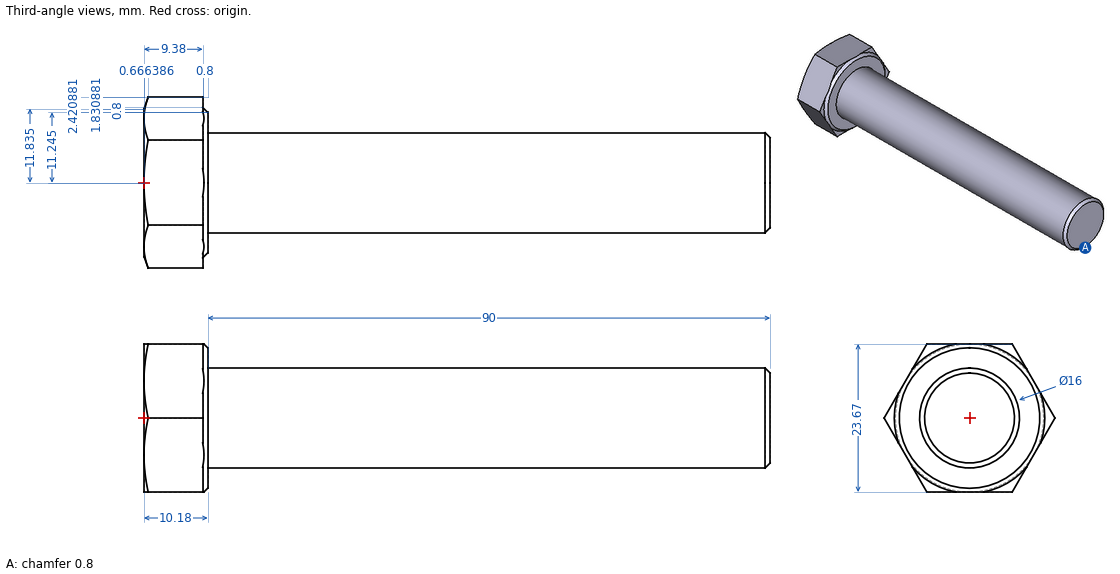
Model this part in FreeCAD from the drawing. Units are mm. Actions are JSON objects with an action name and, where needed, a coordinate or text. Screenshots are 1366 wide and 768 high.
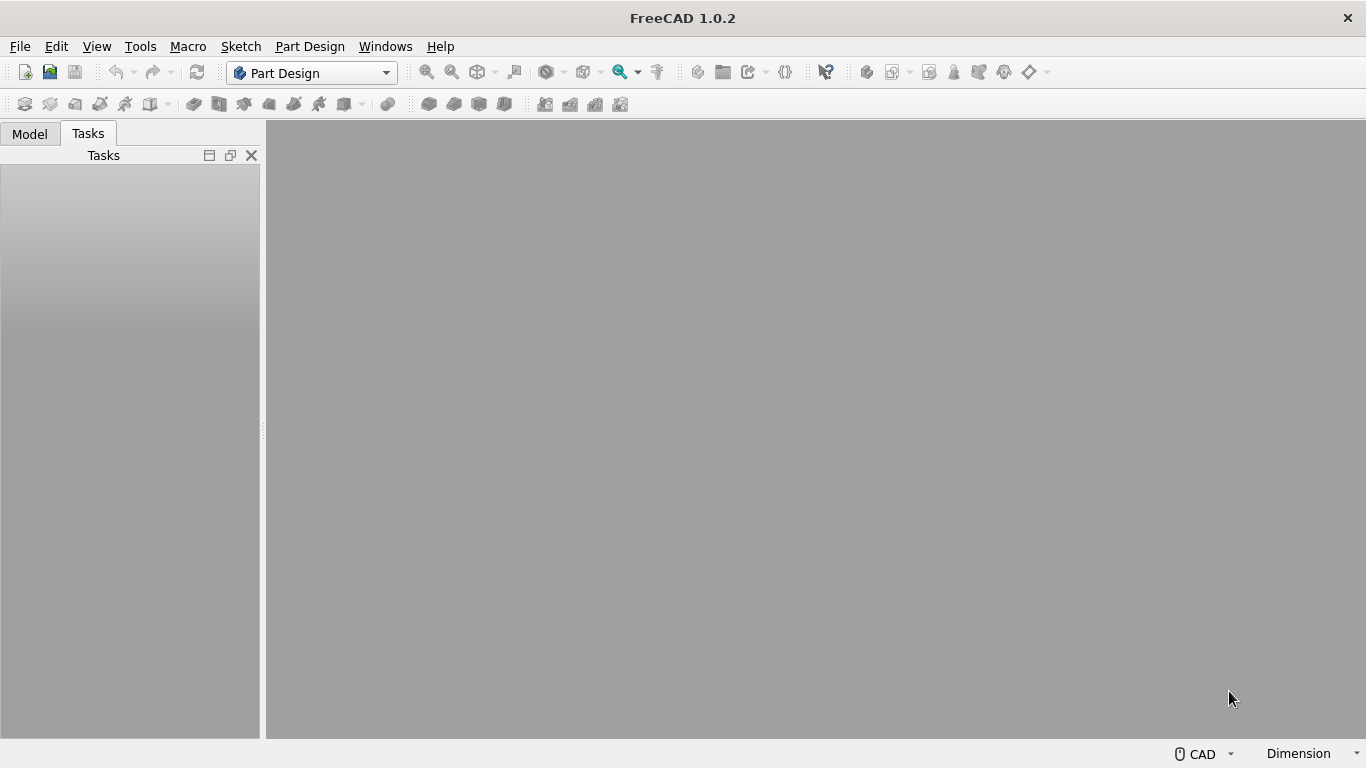
{"action": "key", "text": "ctrl+n"}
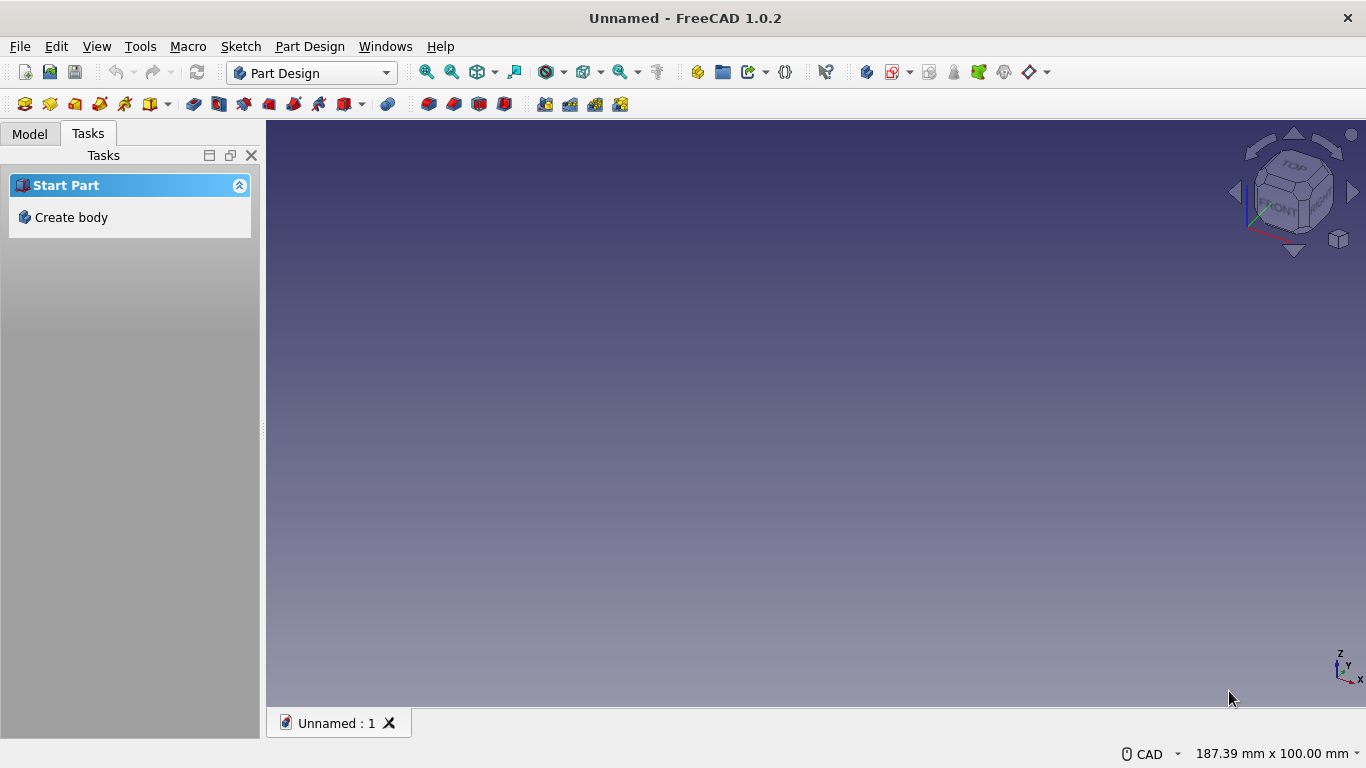
{"action": "left_click", "coordinate": [892, 72]}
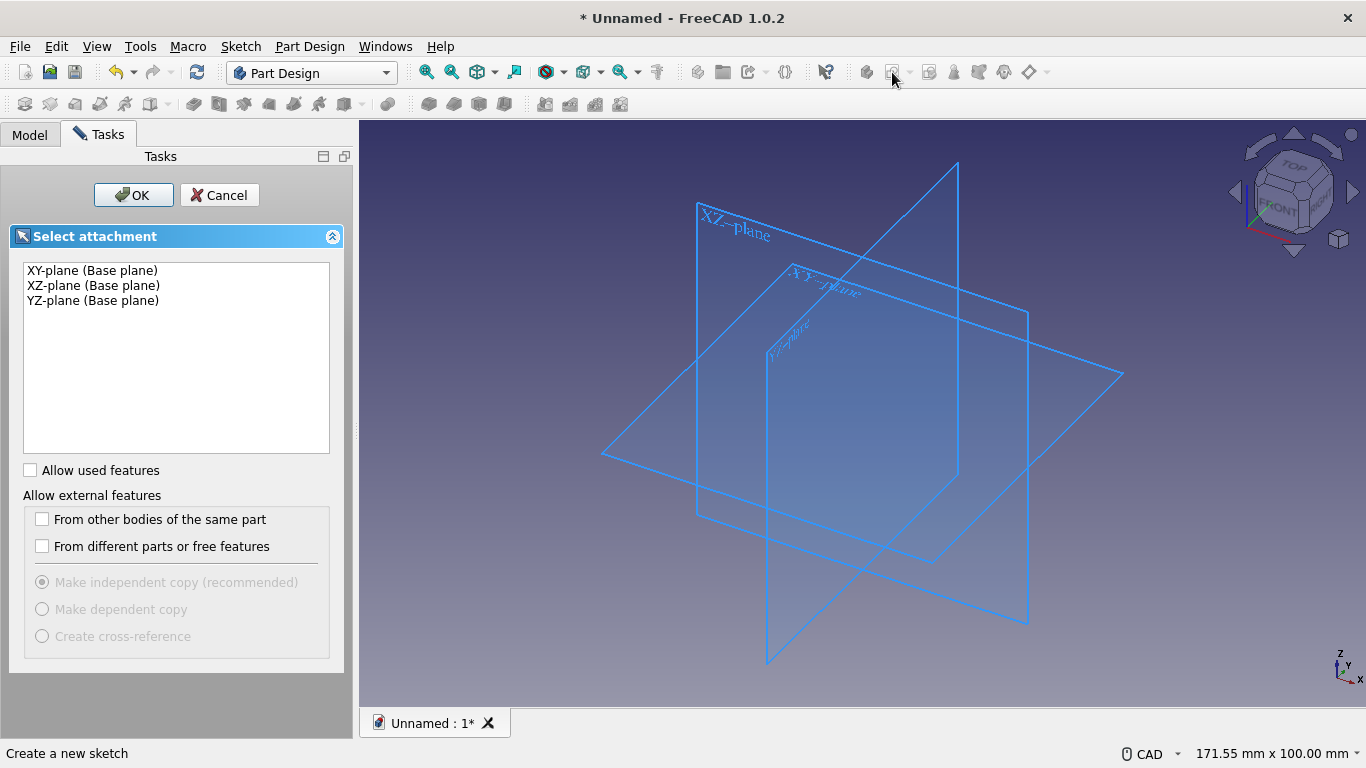
{"action": "left_click", "coordinate": [84, 300]}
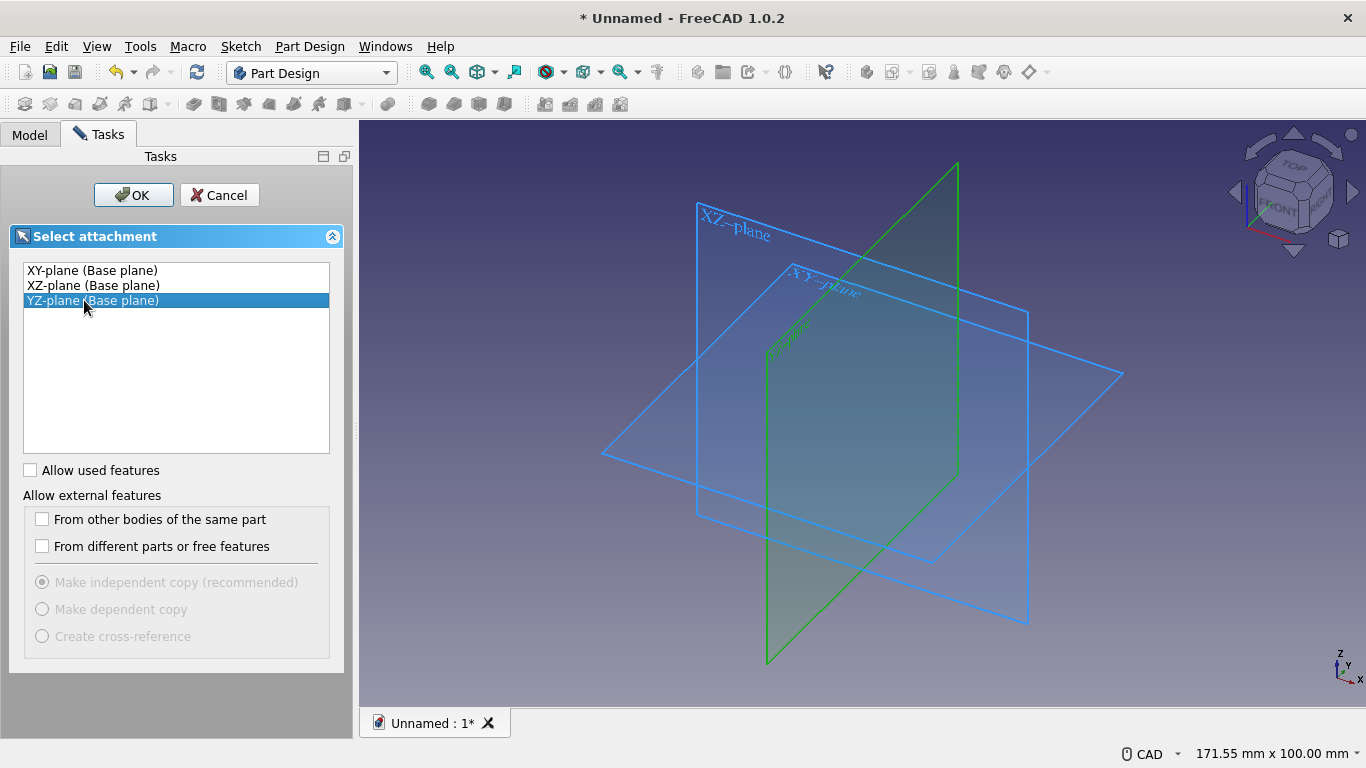
{"action": "left_click", "coordinate": [134, 195]}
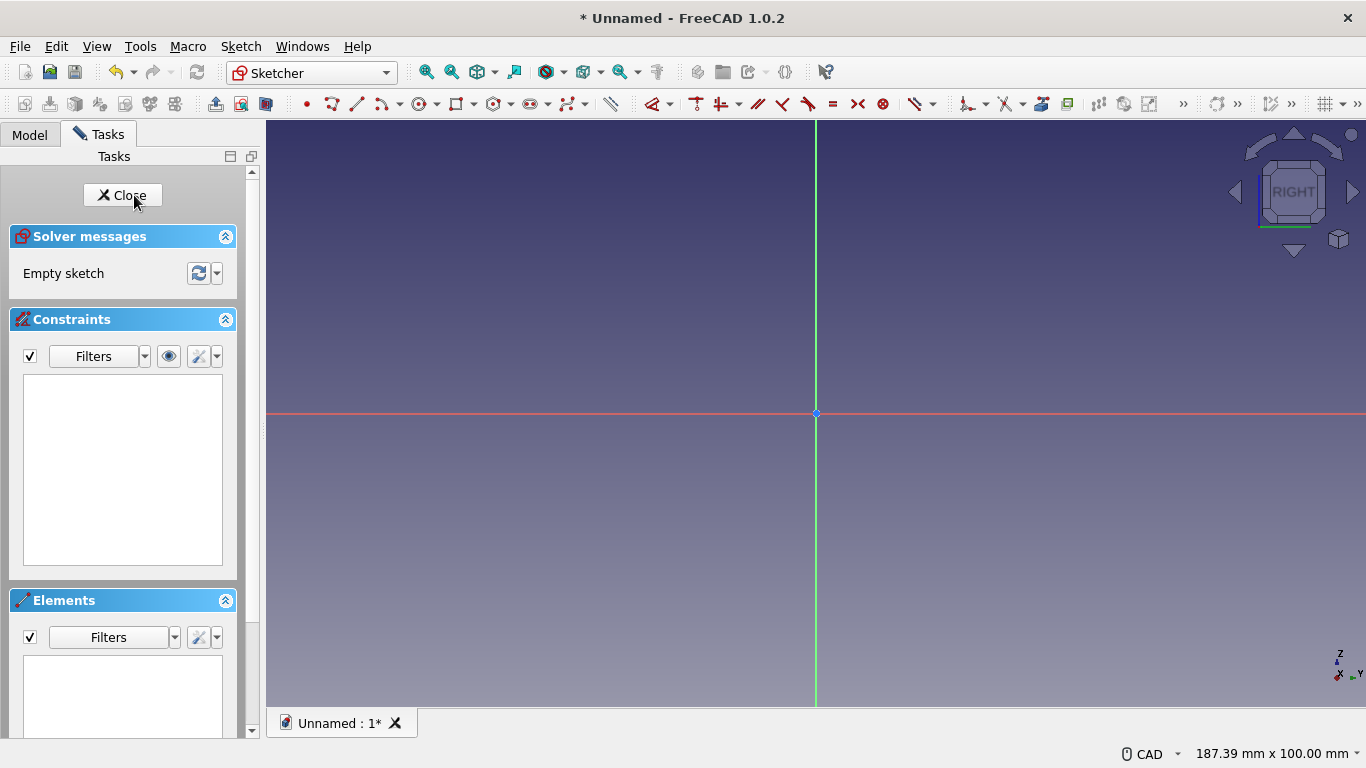
{"action": "scroll", "coordinate": [856, 414], "scroll_direction": "up", "scroll_amount": 5}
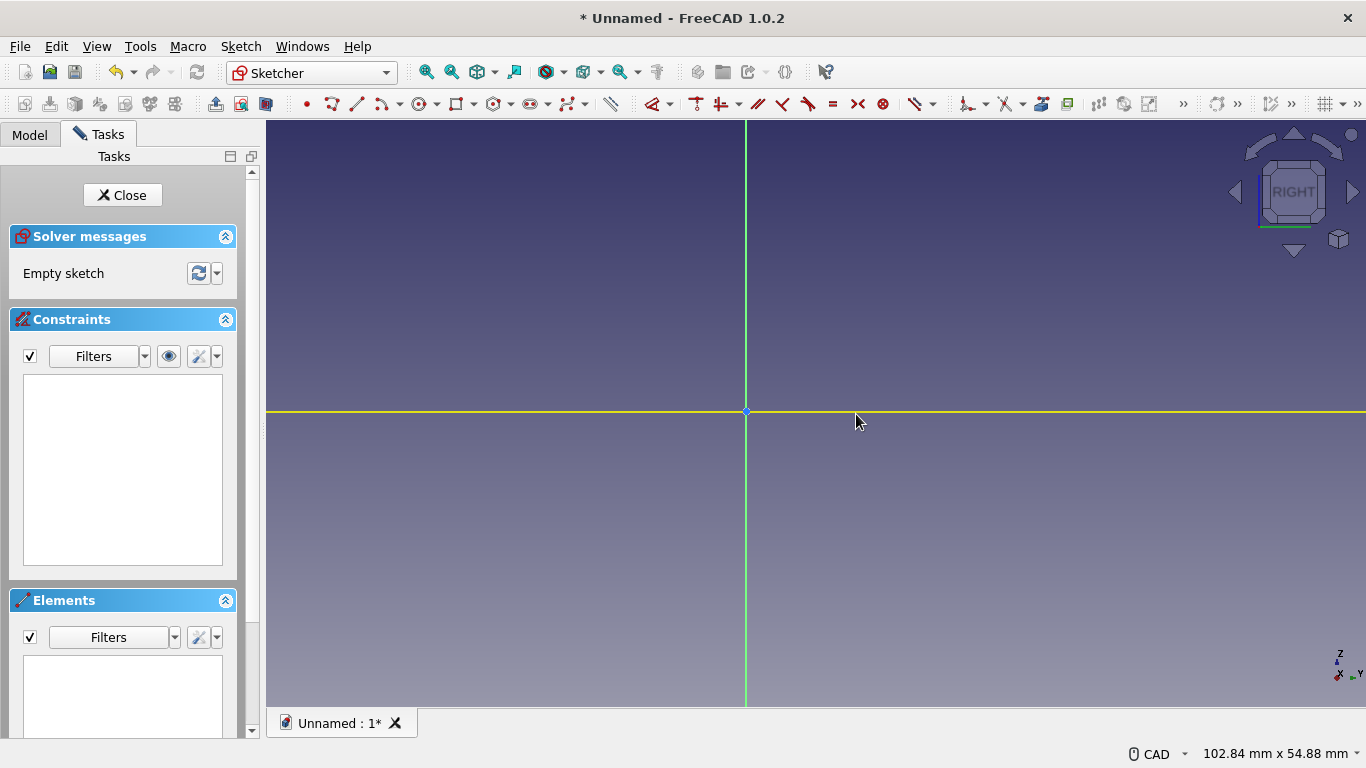
{"action": "left_click", "coordinate": [492, 104]}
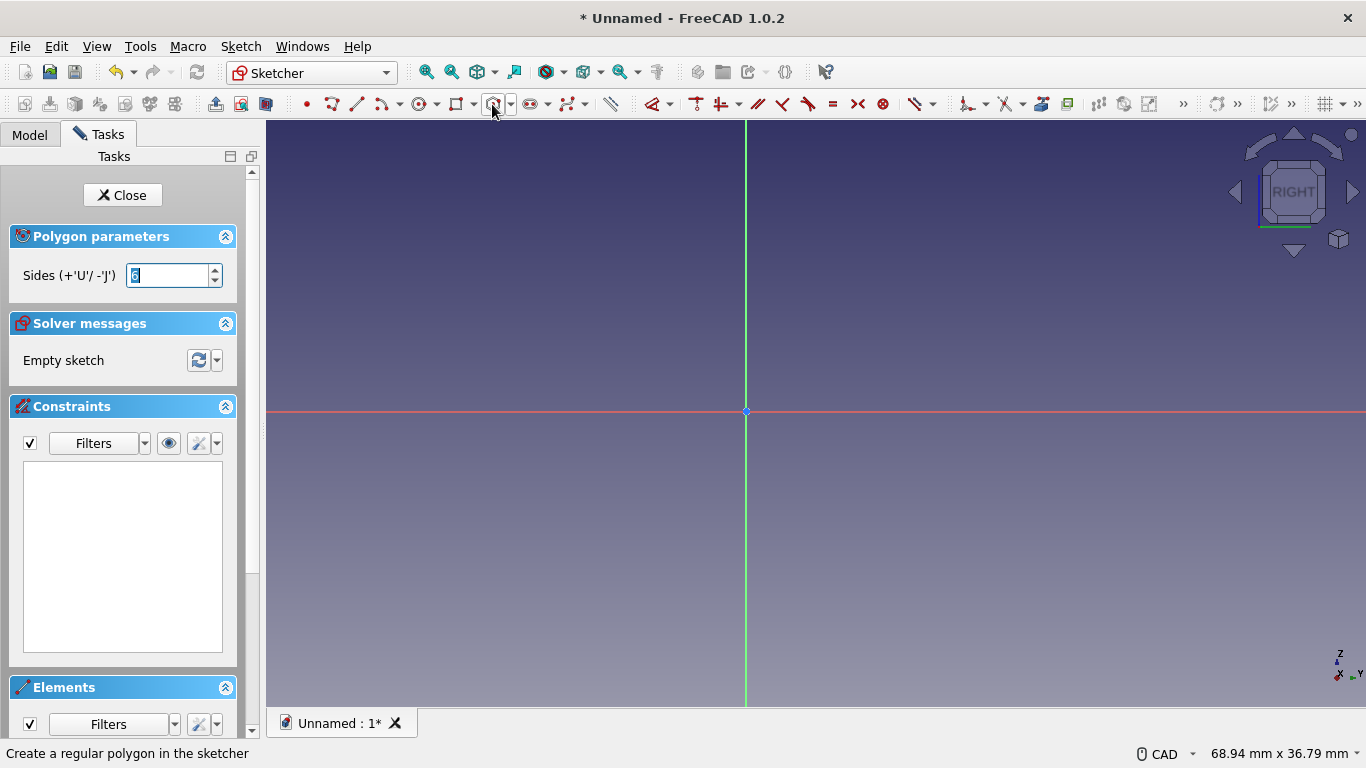
{"action": "left_click", "coordinate": [746, 412]}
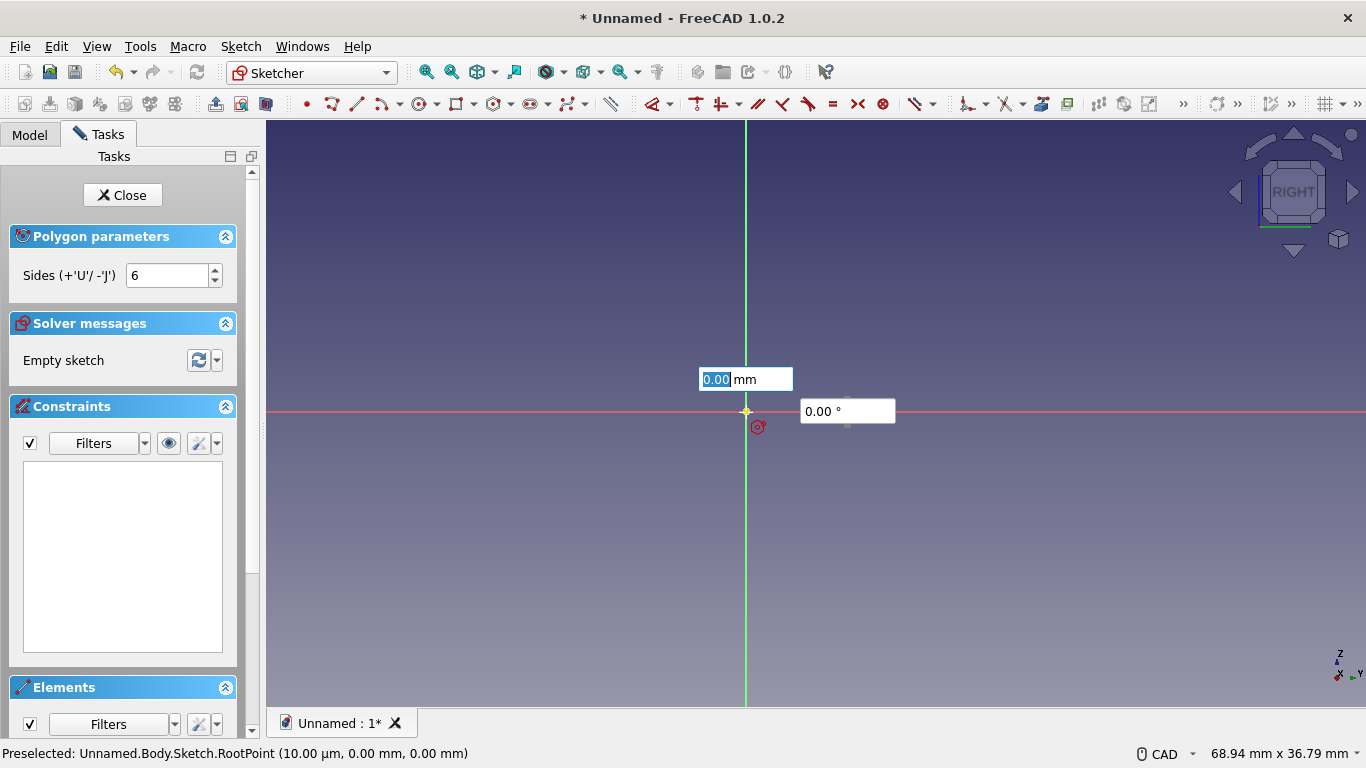
{"action": "left_click", "coordinate": [964, 412]}
{"action": "right_click", "coordinate": [964, 412]}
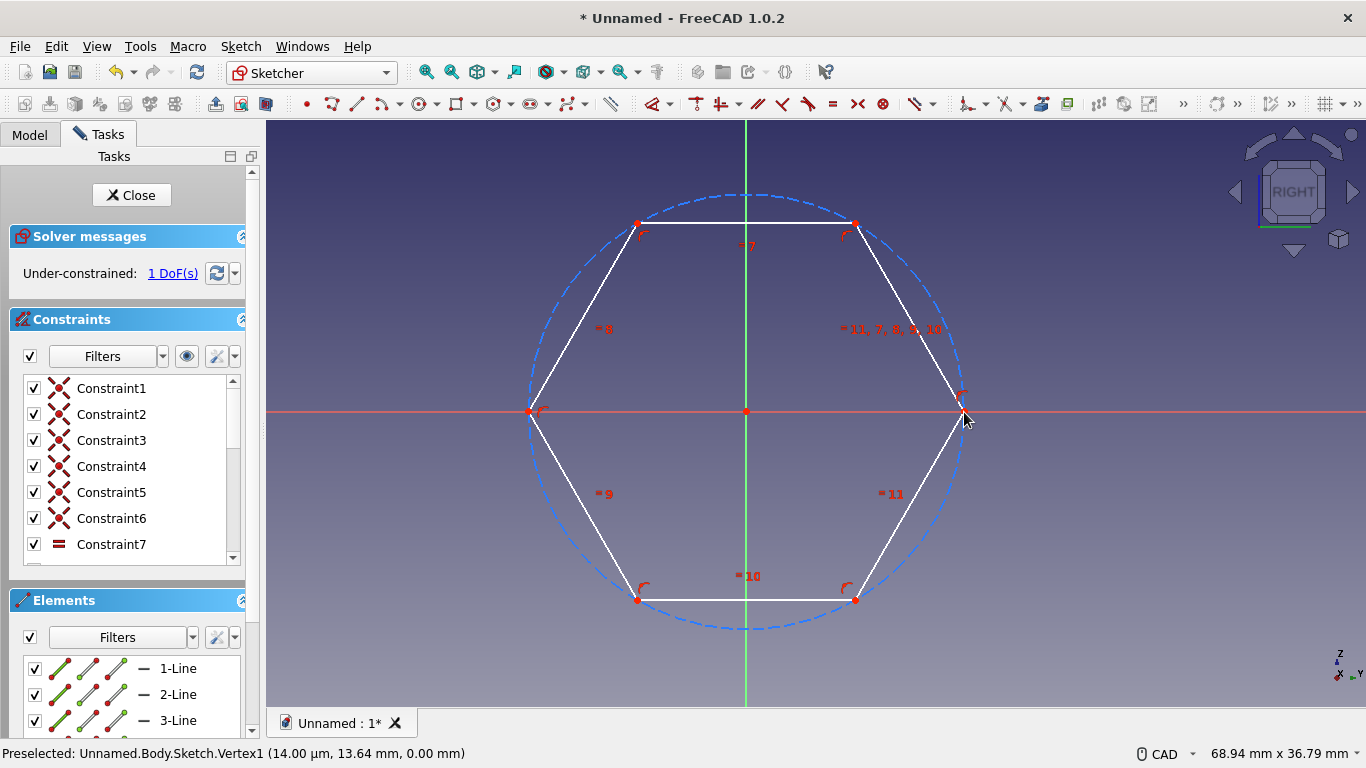
{"action": "left_click", "coordinate": [638, 600]}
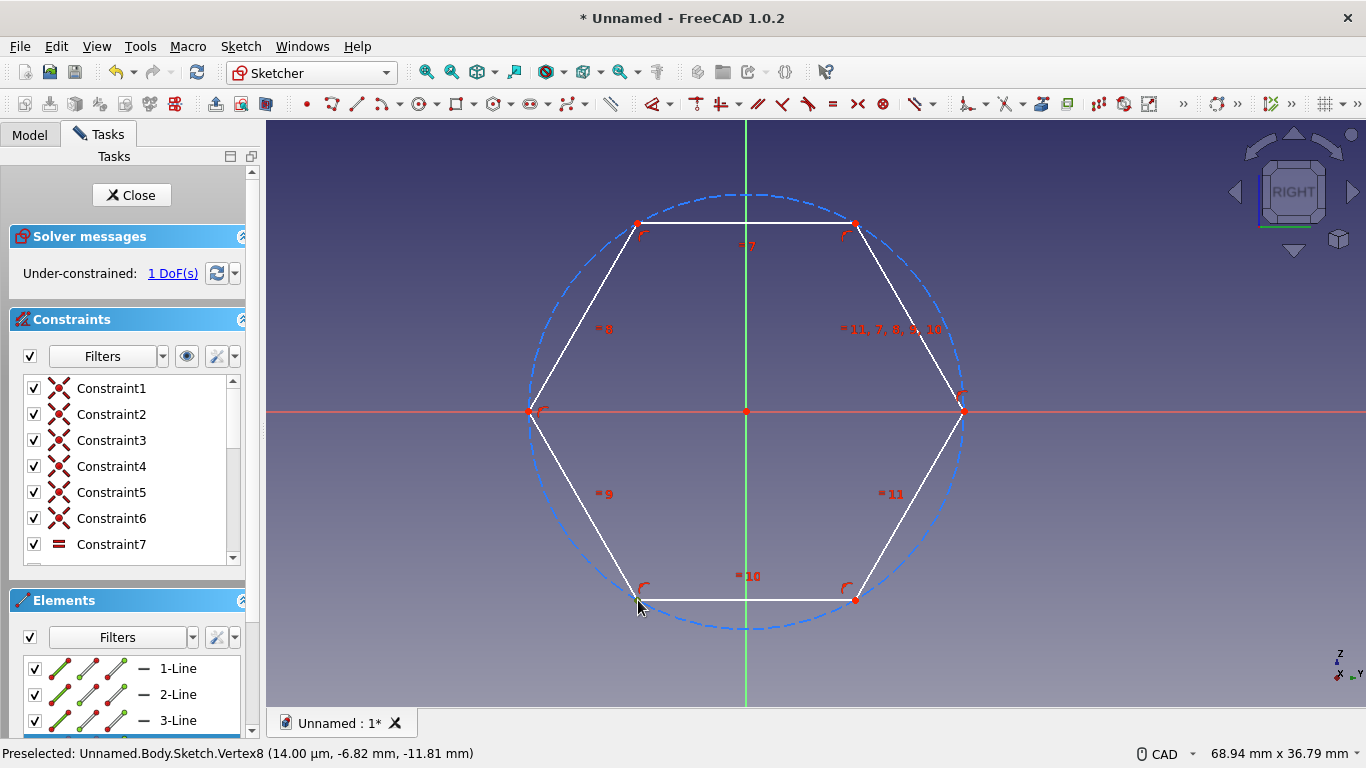
{"action": "left_click", "coordinate": [855, 223]}